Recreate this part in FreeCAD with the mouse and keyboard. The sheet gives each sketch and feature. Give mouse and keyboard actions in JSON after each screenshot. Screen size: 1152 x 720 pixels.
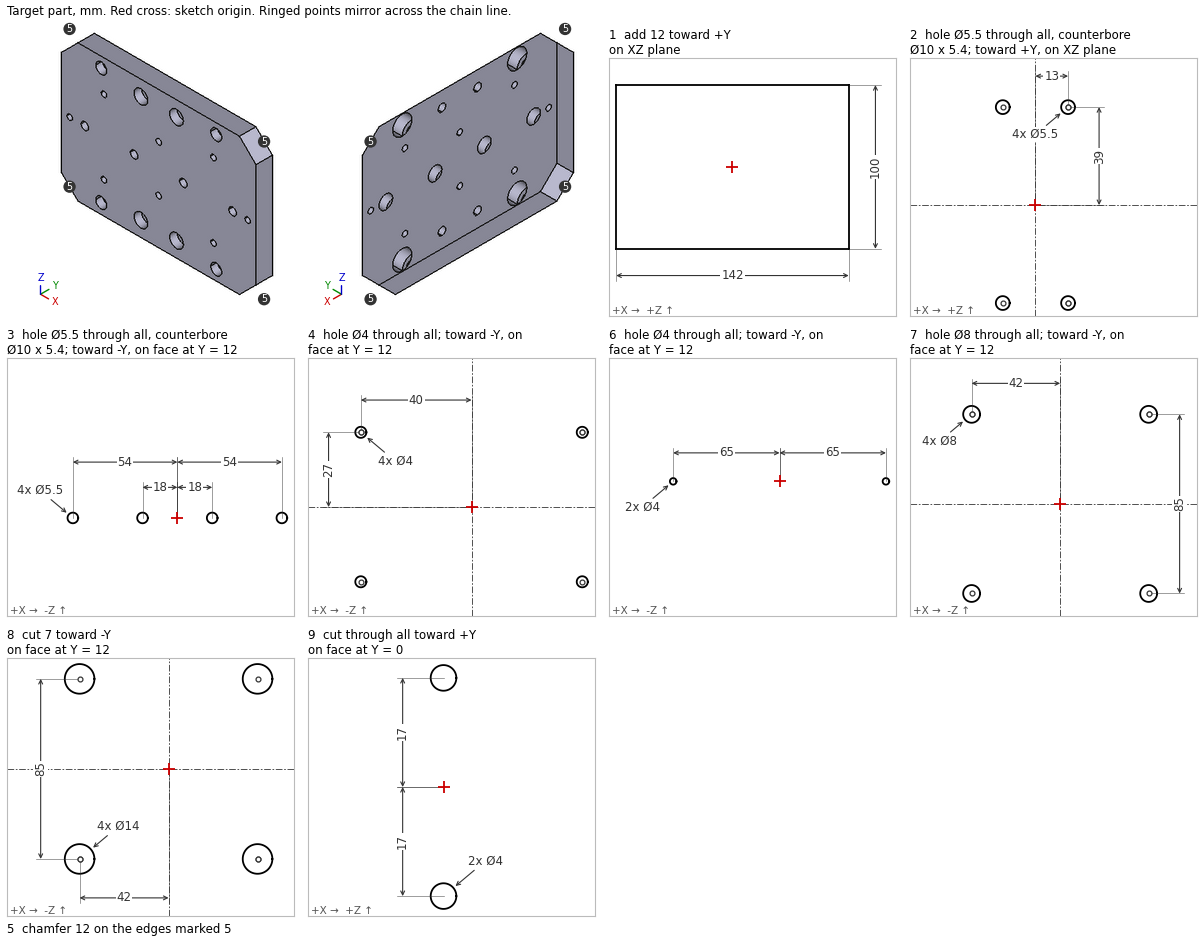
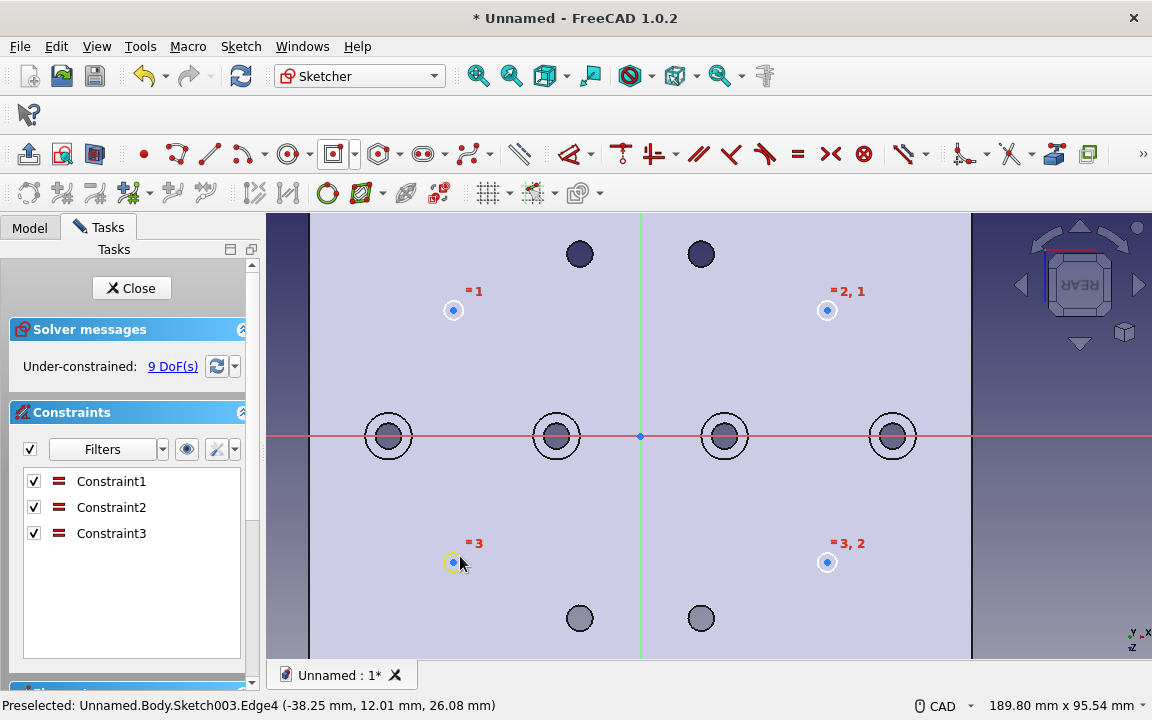
{"action": "left_click", "coordinate": [454, 310]}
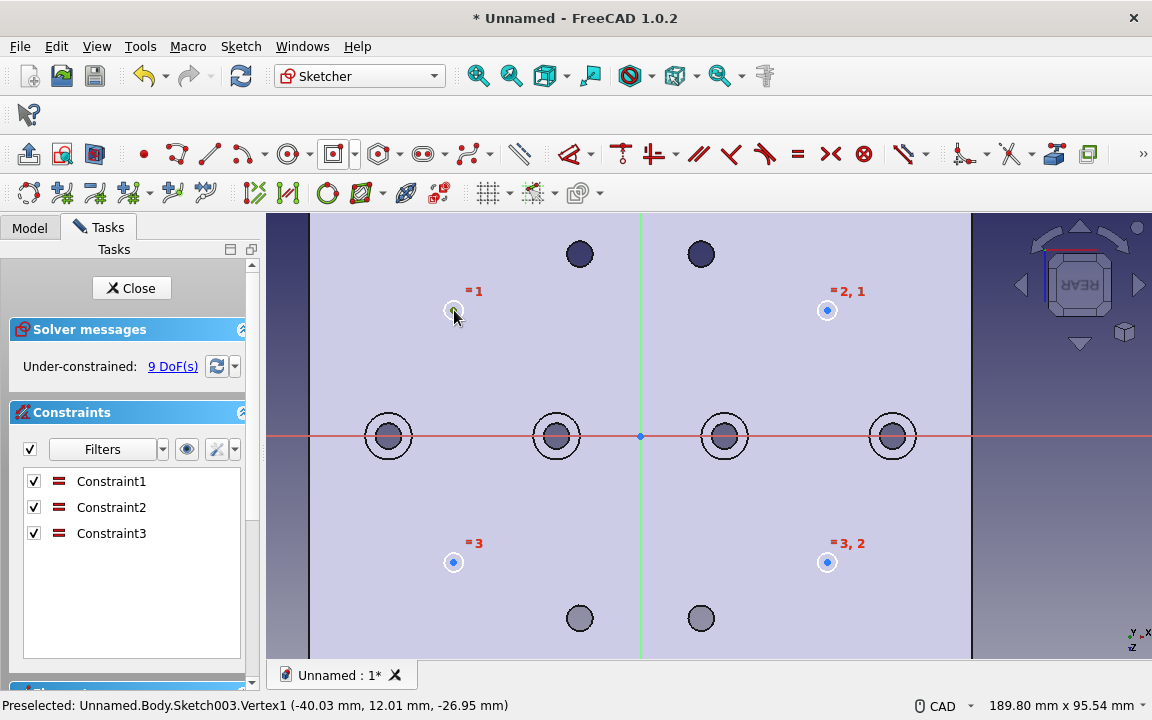
{"action": "left_click", "coordinate": [827, 311]}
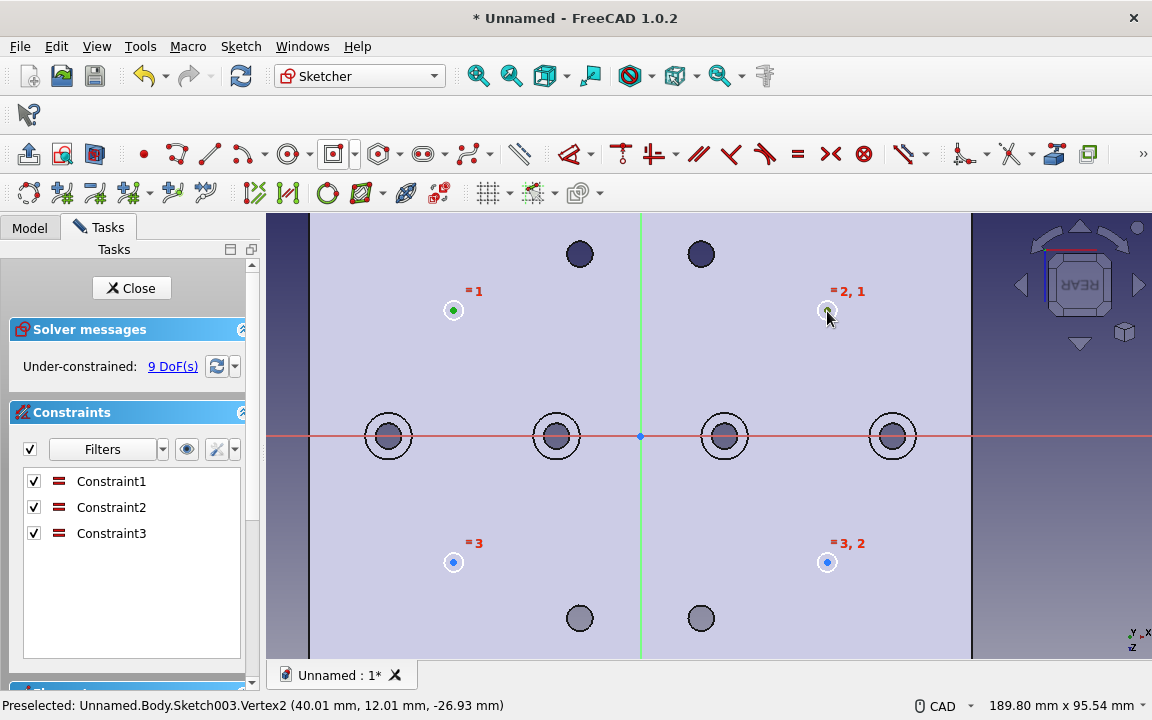
{"action": "left_click", "coordinate": [641, 603]}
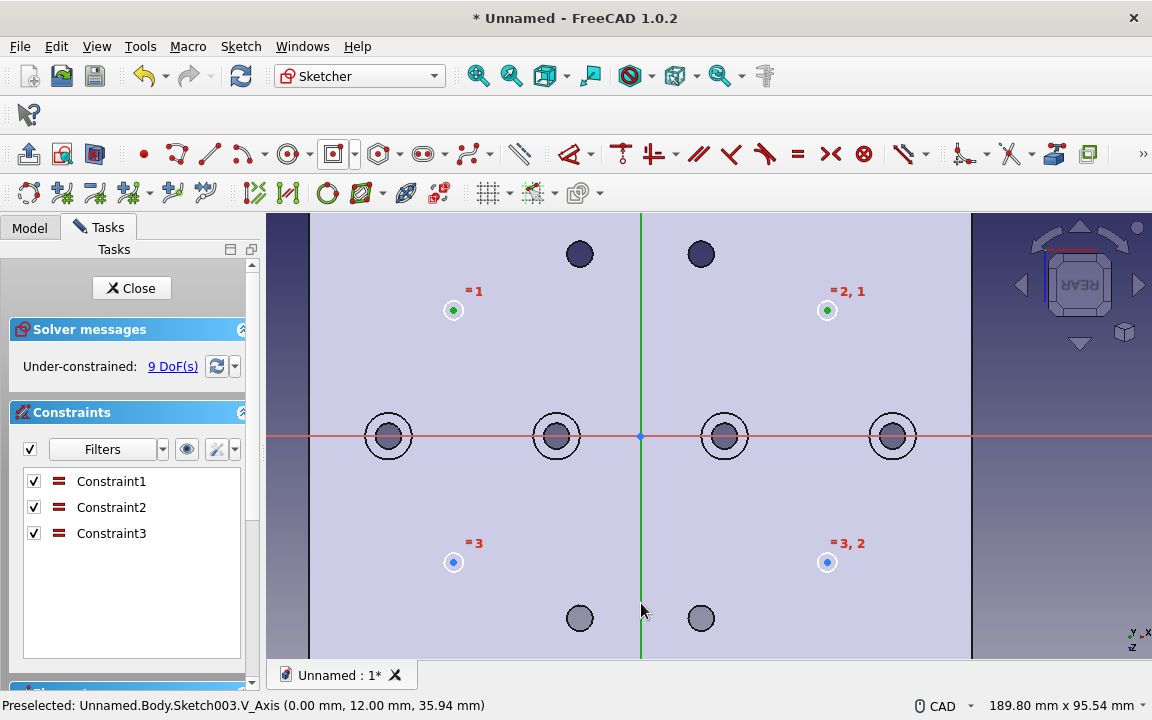
{"action": "left_click", "coordinate": [831, 154]}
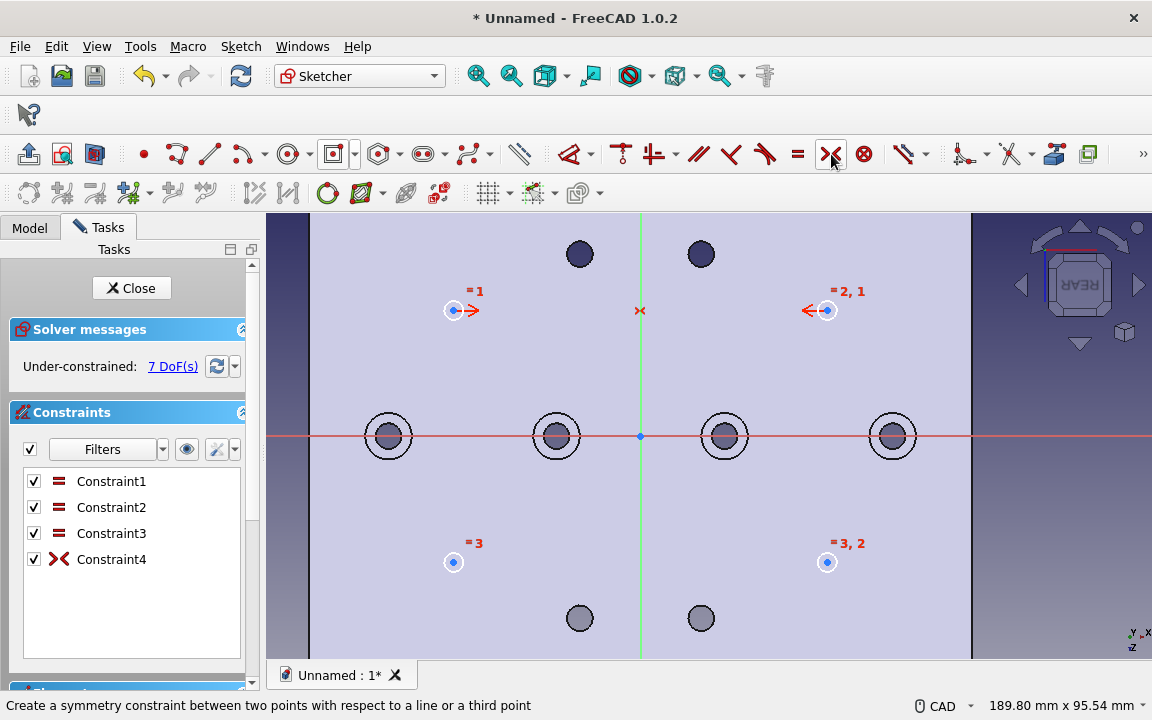
{"action": "left_click", "coordinate": [827, 311]}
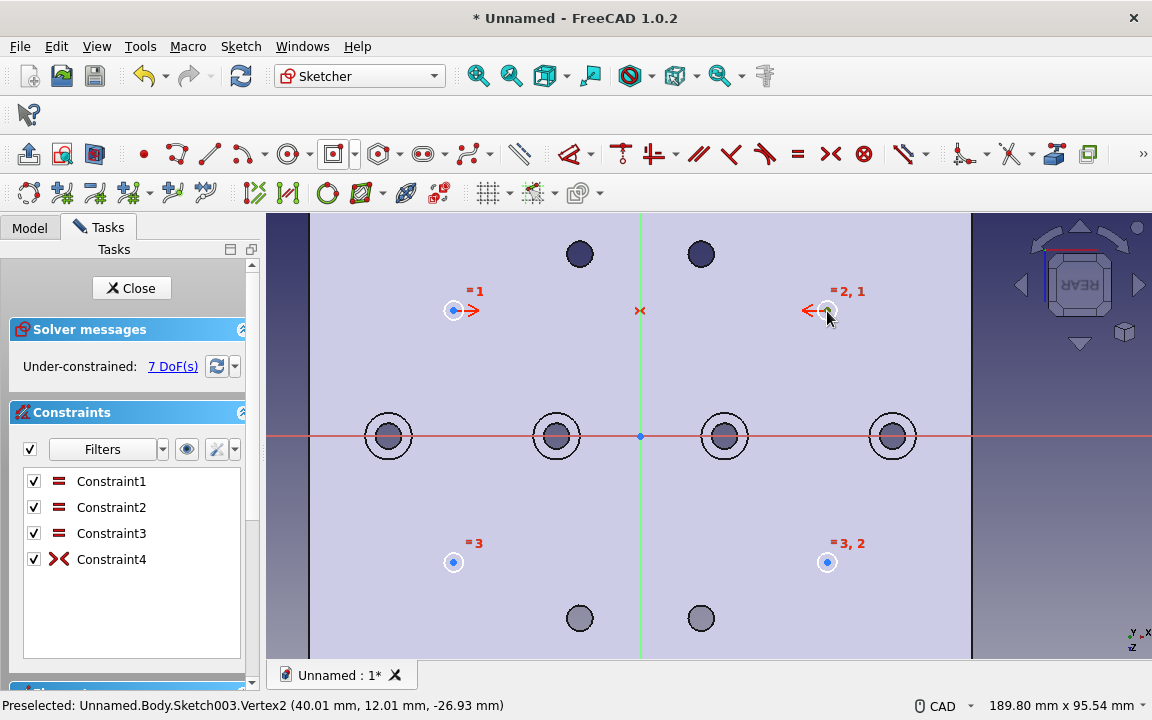
{"action": "left_click", "coordinate": [827, 562]}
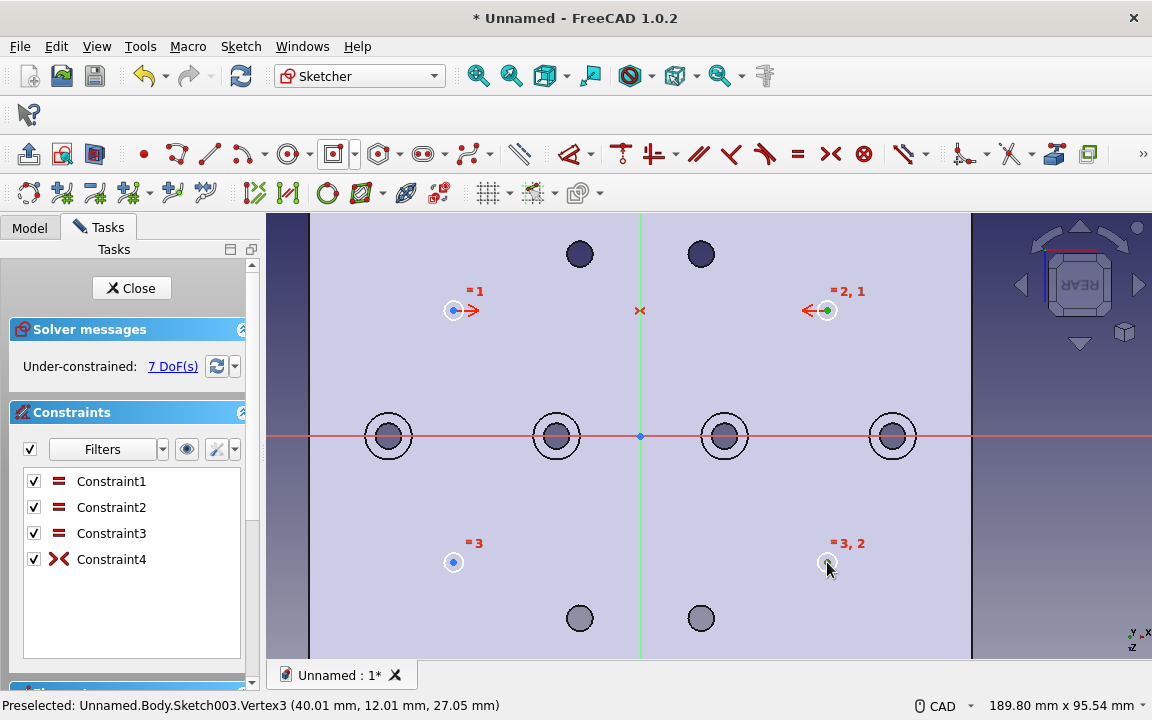
{"action": "left_click", "coordinate": [344, 436]}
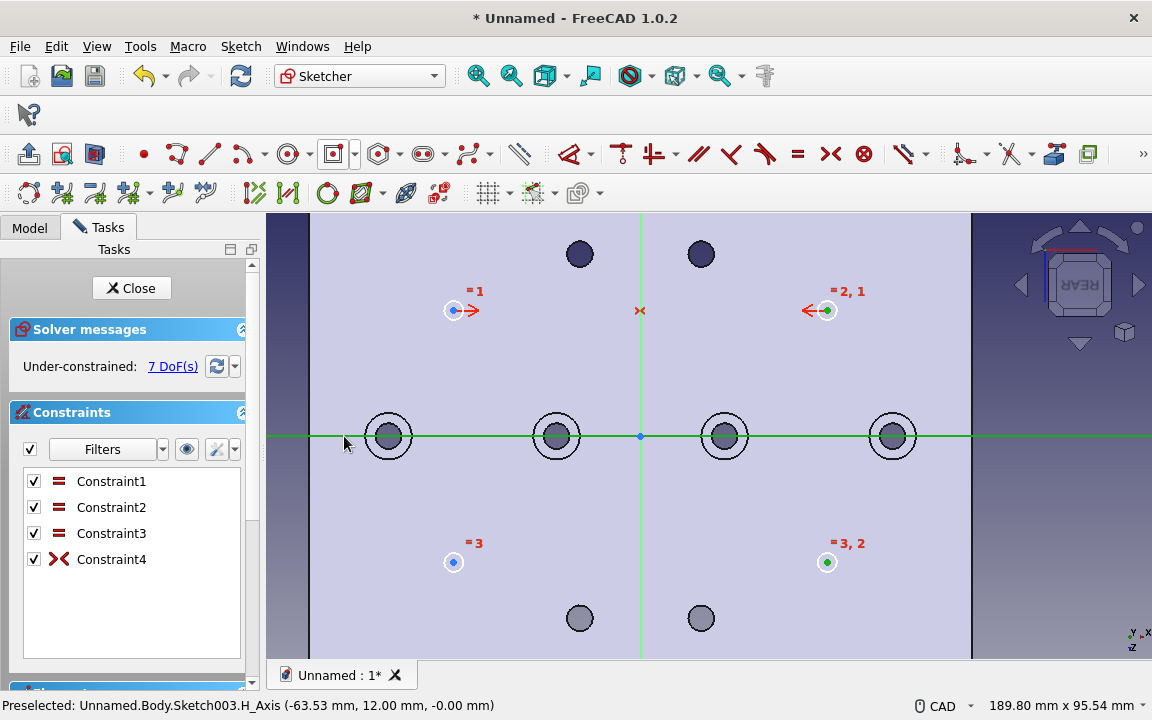
{"action": "left_click", "coordinate": [831, 154]}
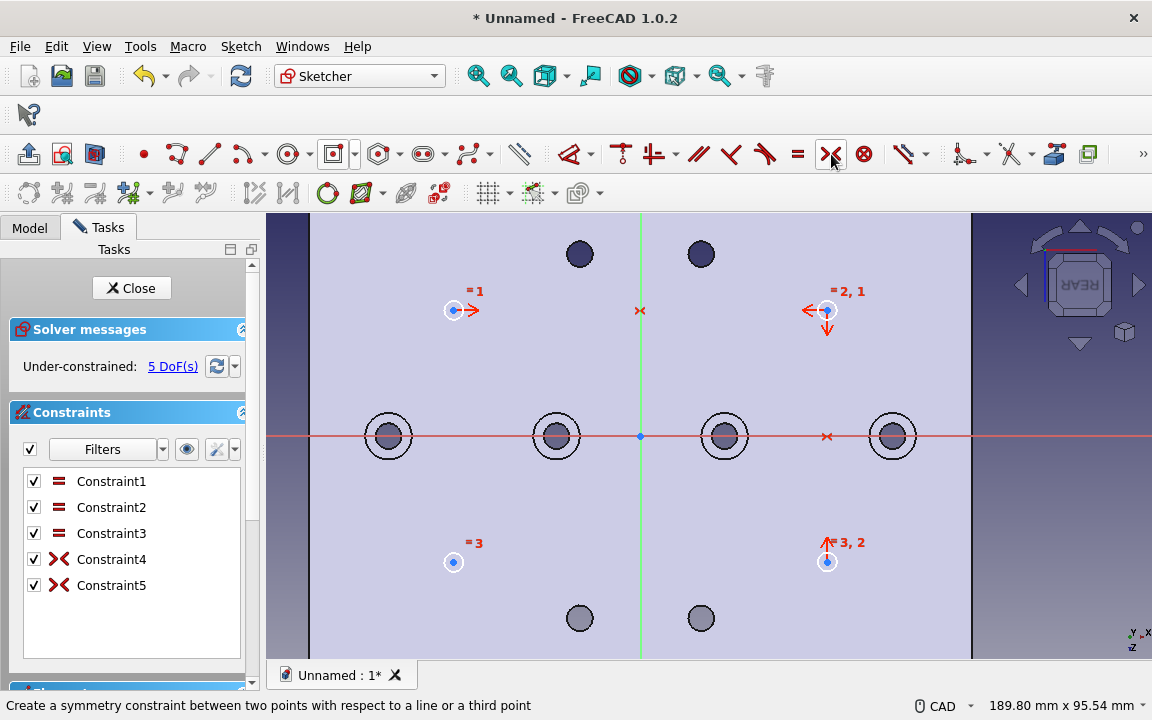
{"action": "left_click", "coordinate": [454, 310]}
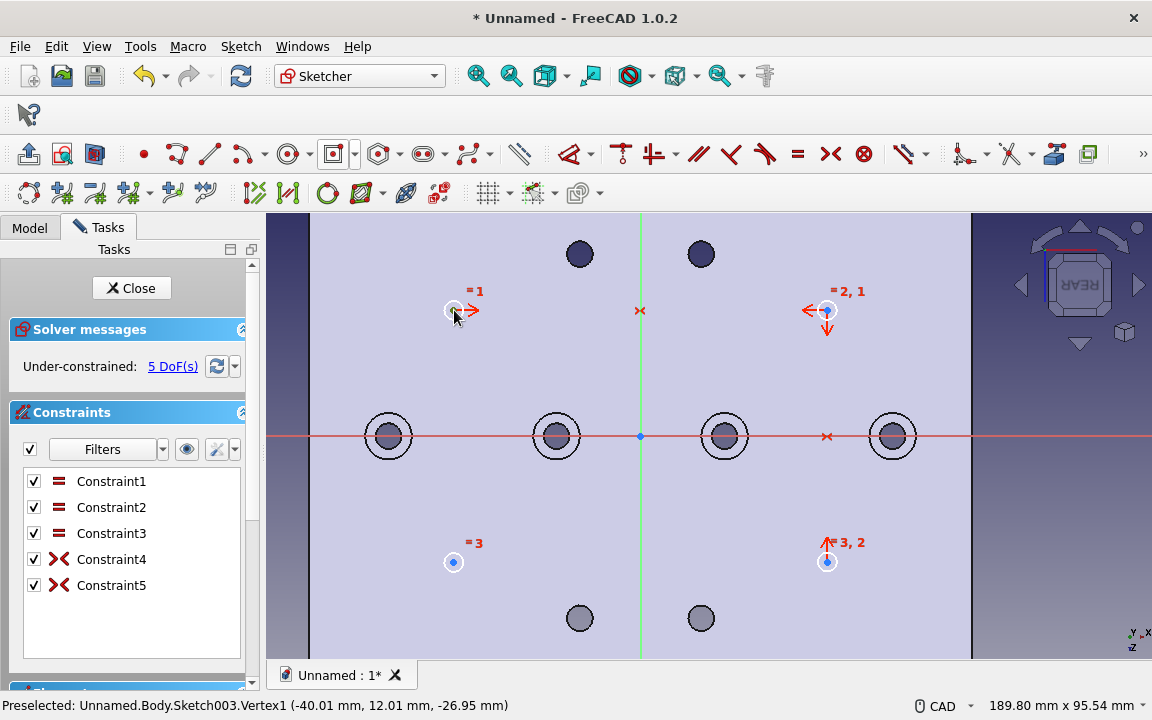
{"action": "left_click", "coordinate": [454, 562]}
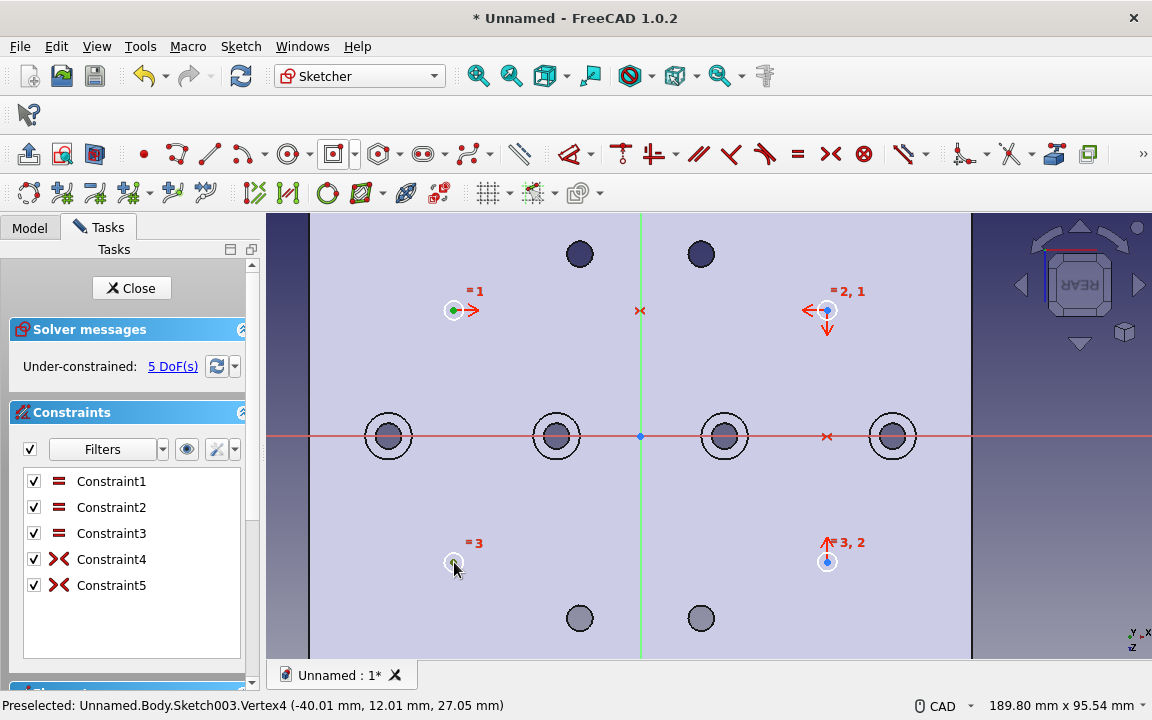
{"action": "left_click", "coordinate": [344, 436]}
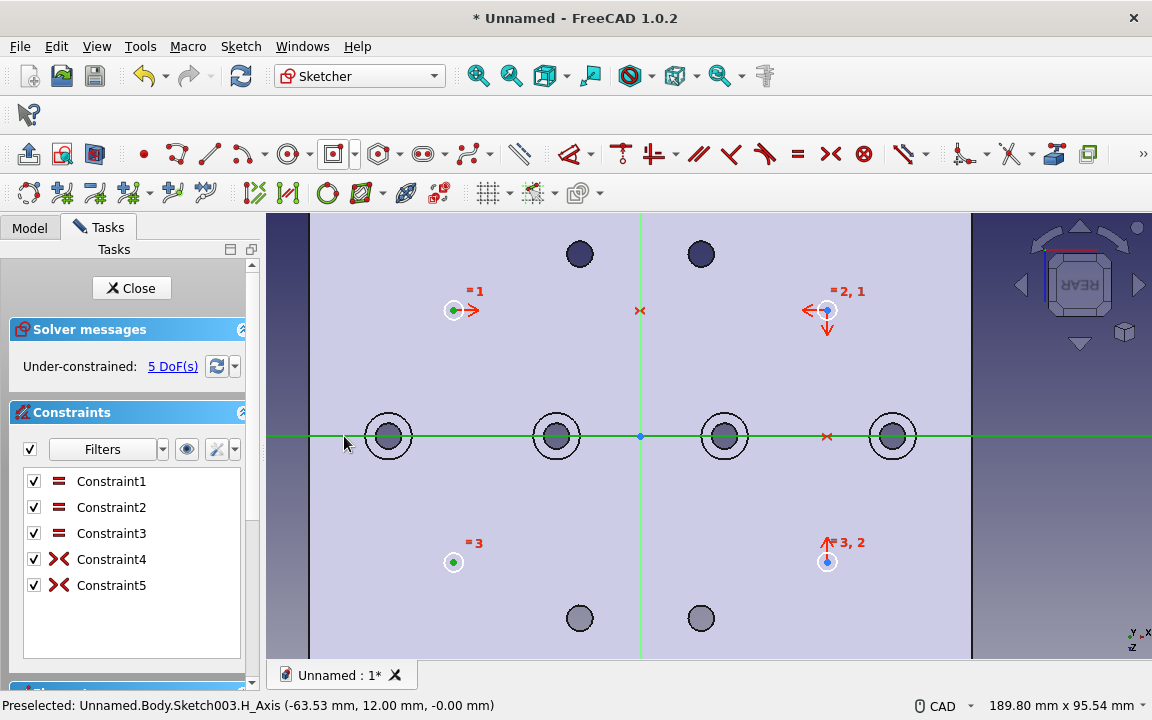
{"action": "left_click", "coordinate": [831, 154]}